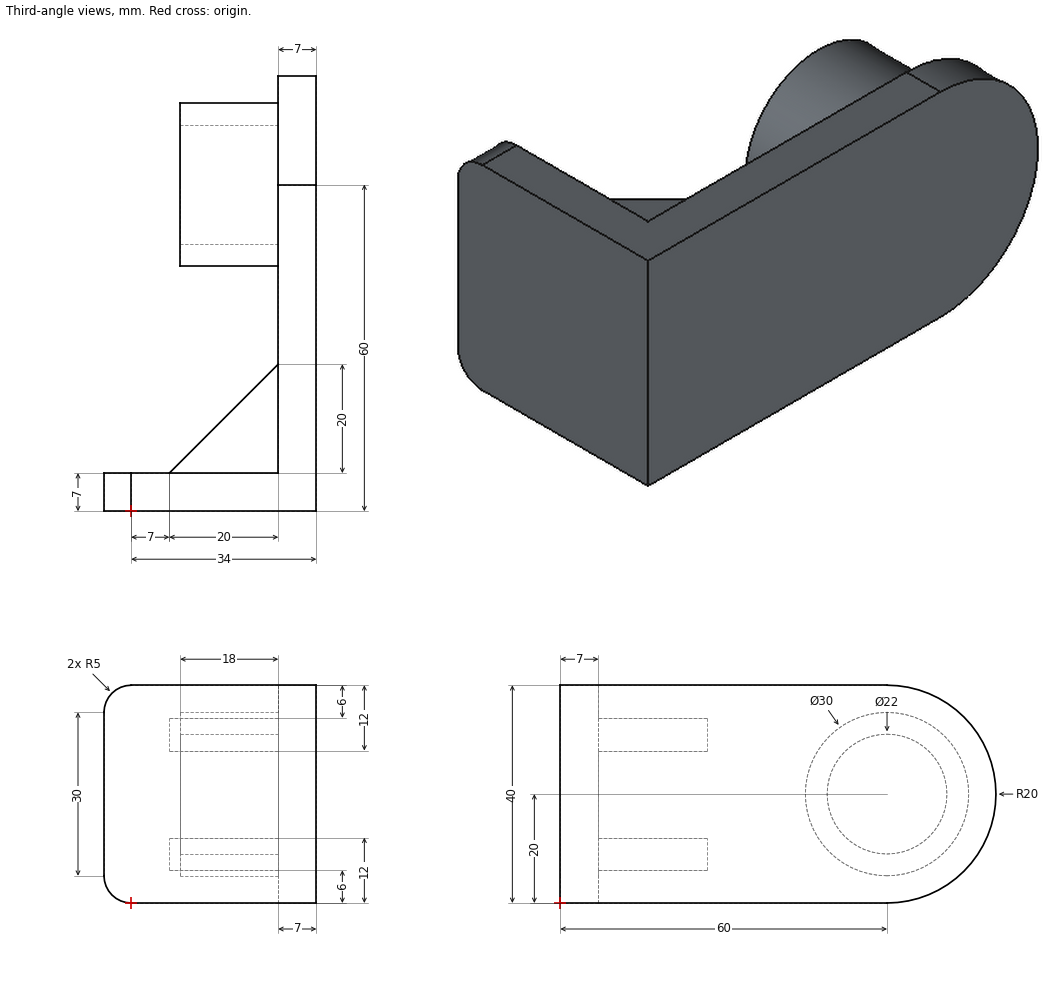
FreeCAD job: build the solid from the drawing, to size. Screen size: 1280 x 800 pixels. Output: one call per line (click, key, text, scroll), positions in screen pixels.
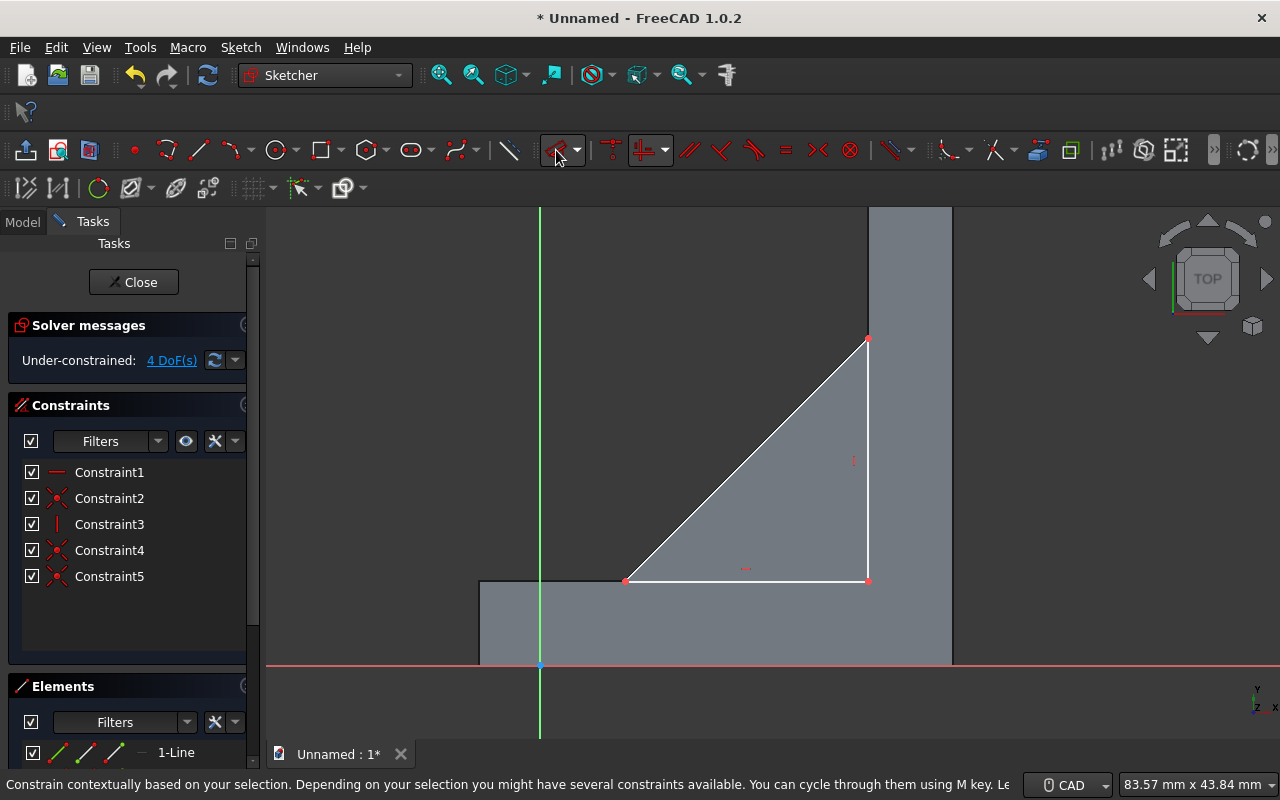
click(698, 582)
click(747, 616)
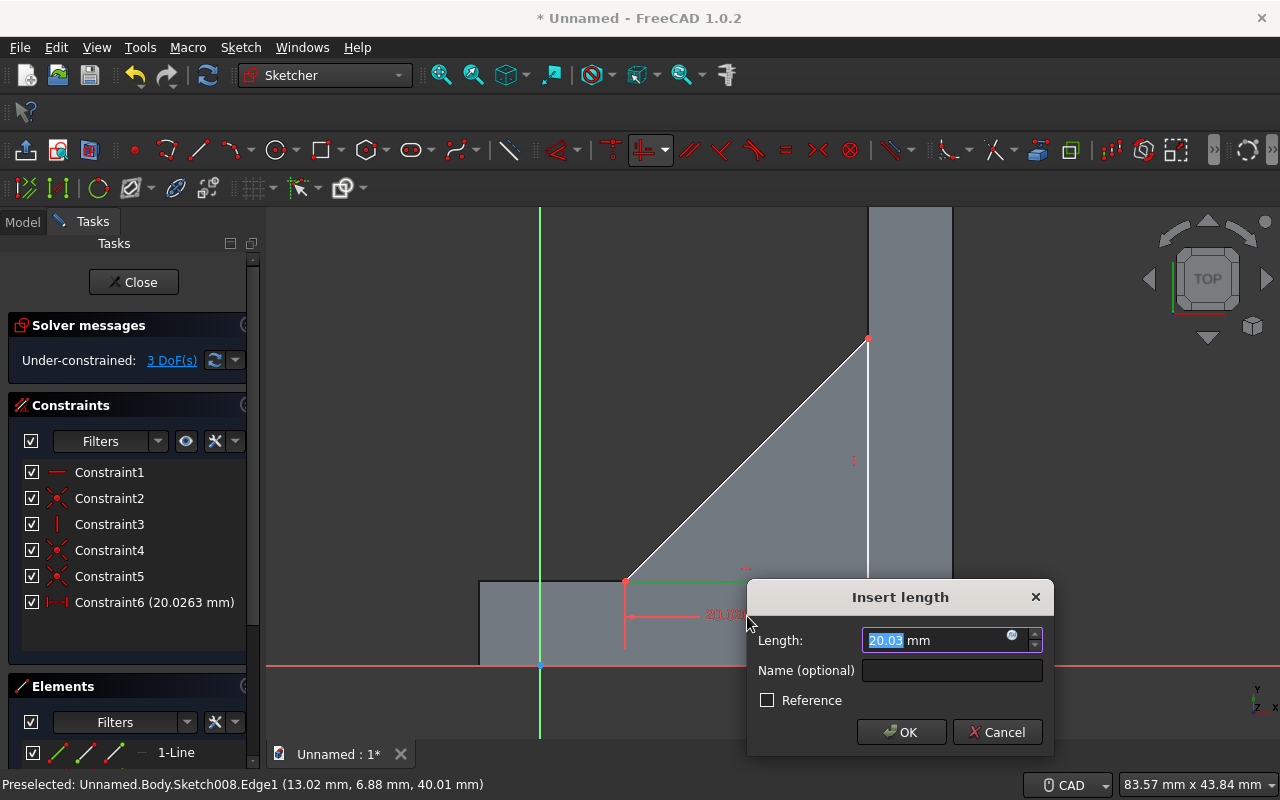
text(20)
key(Return)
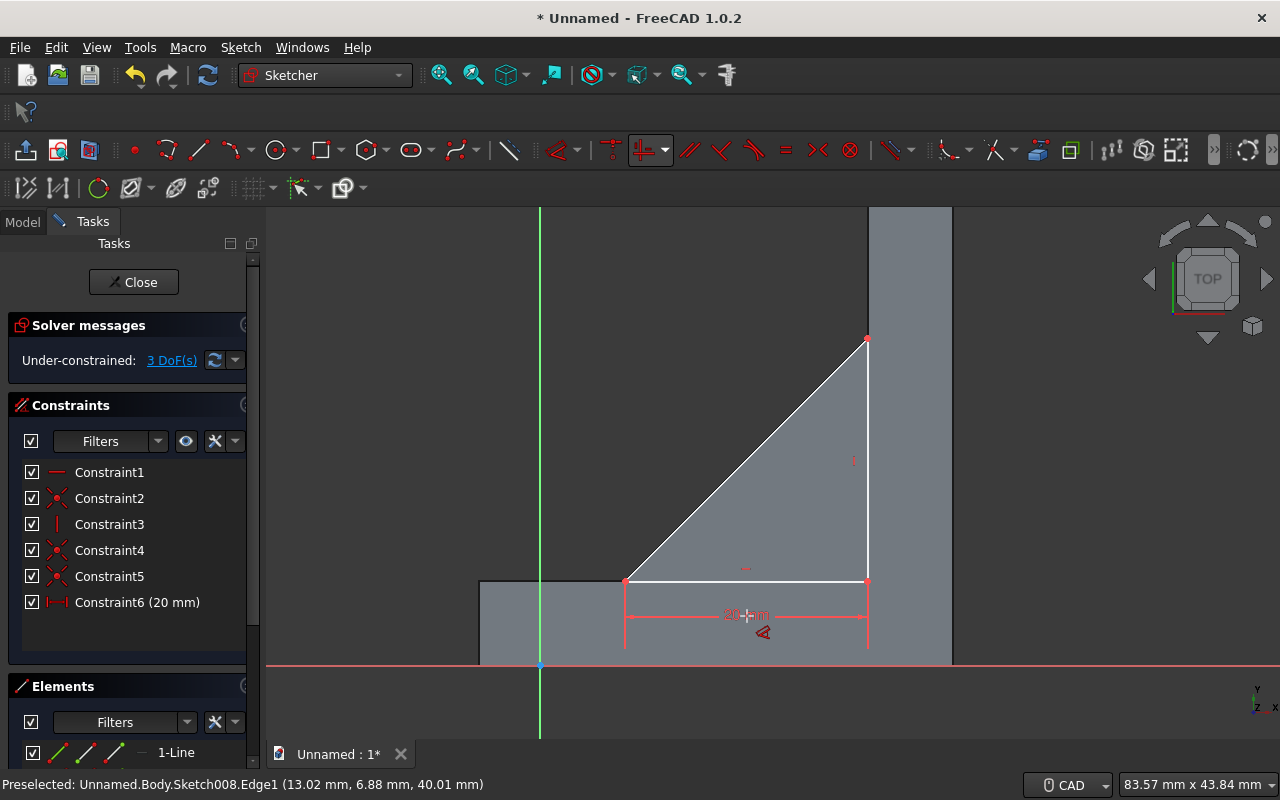
click(868, 509)
click(902, 461)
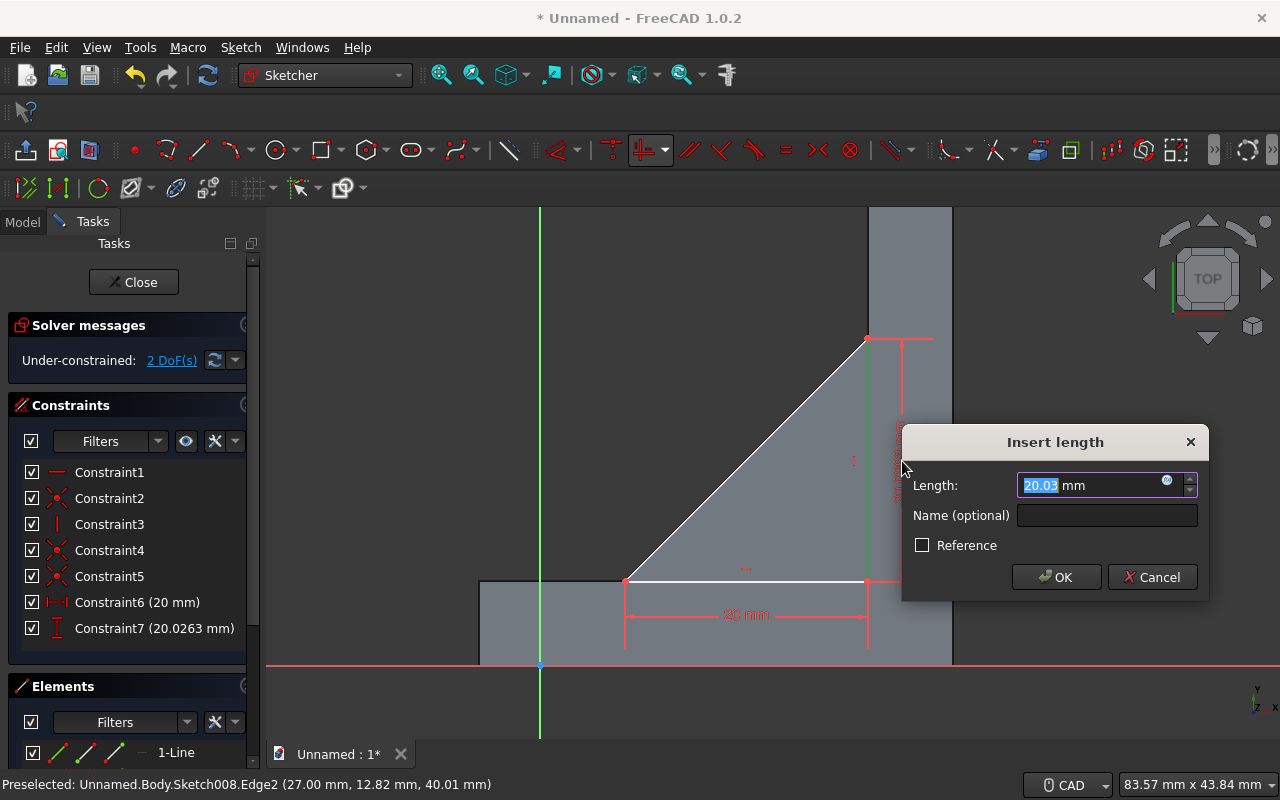
text(20)
key(Return)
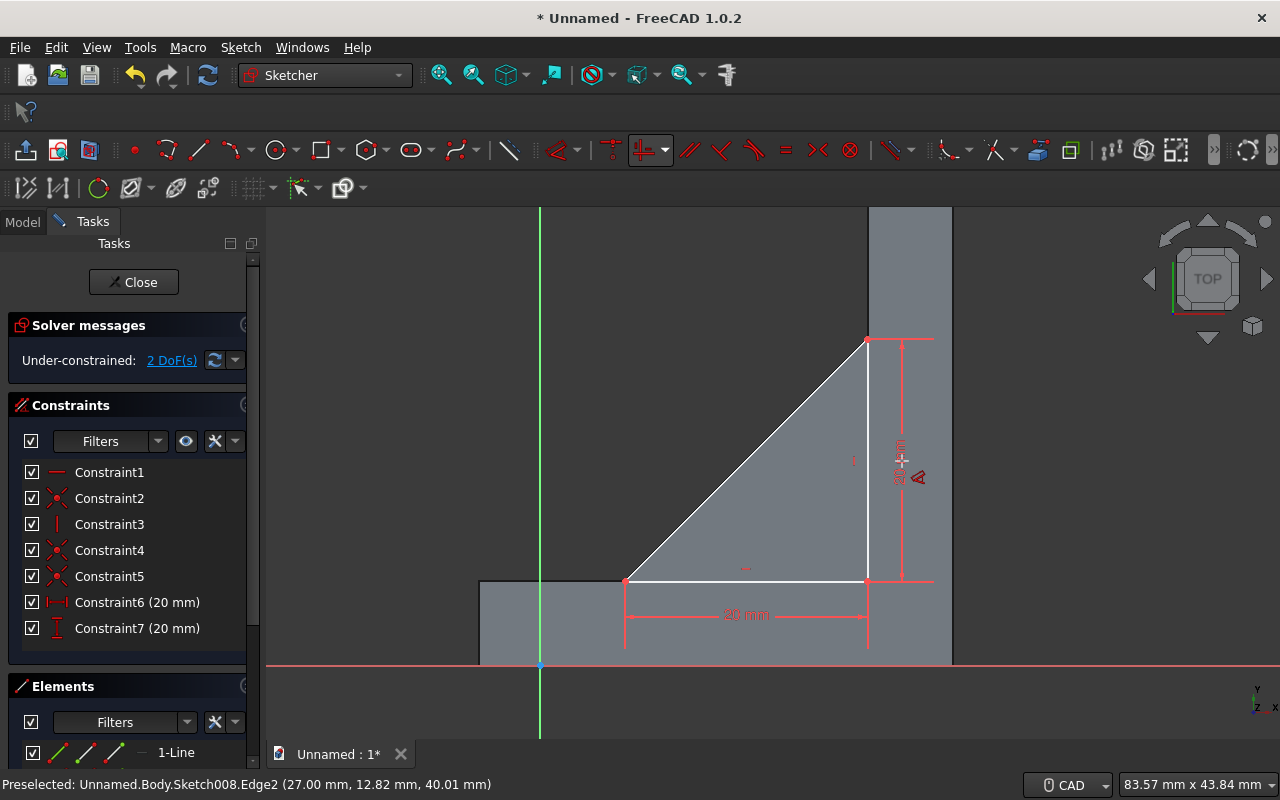
click(625, 582)
click(583, 700)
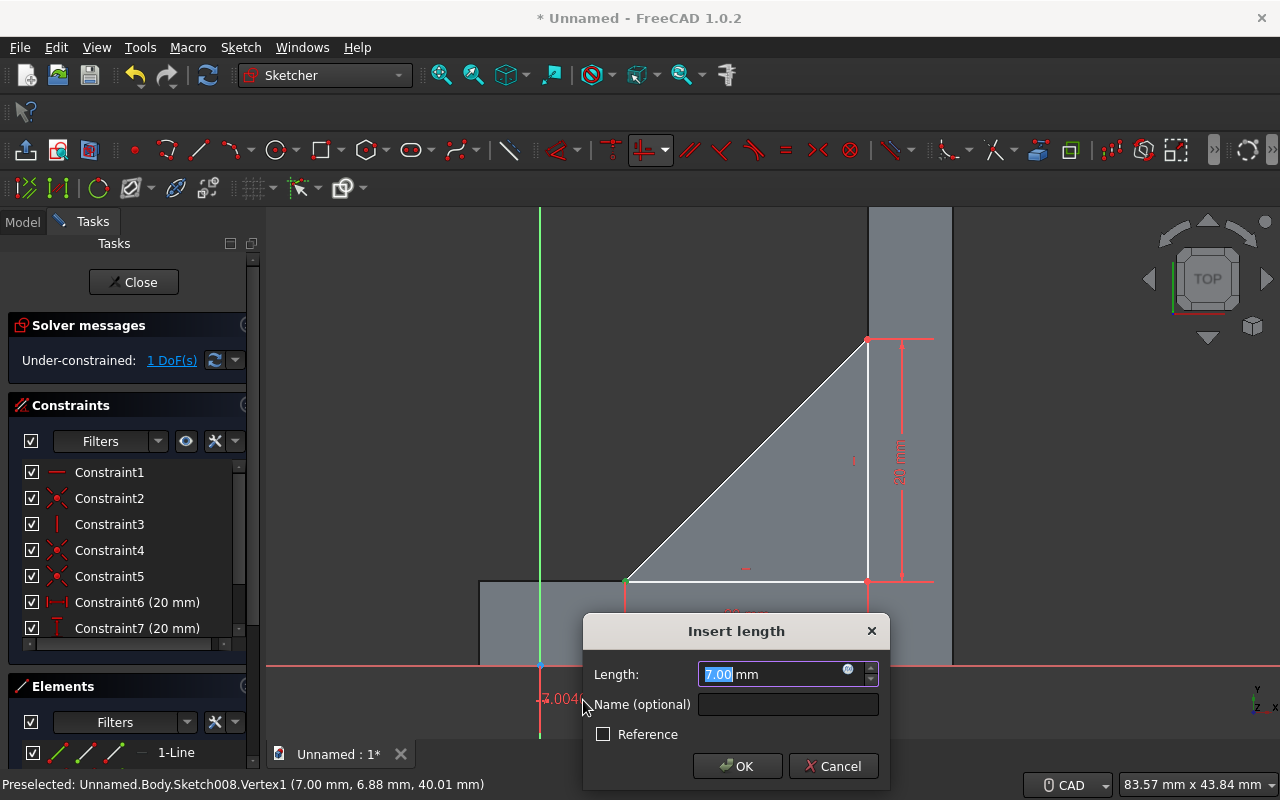
text(7)
key(Return)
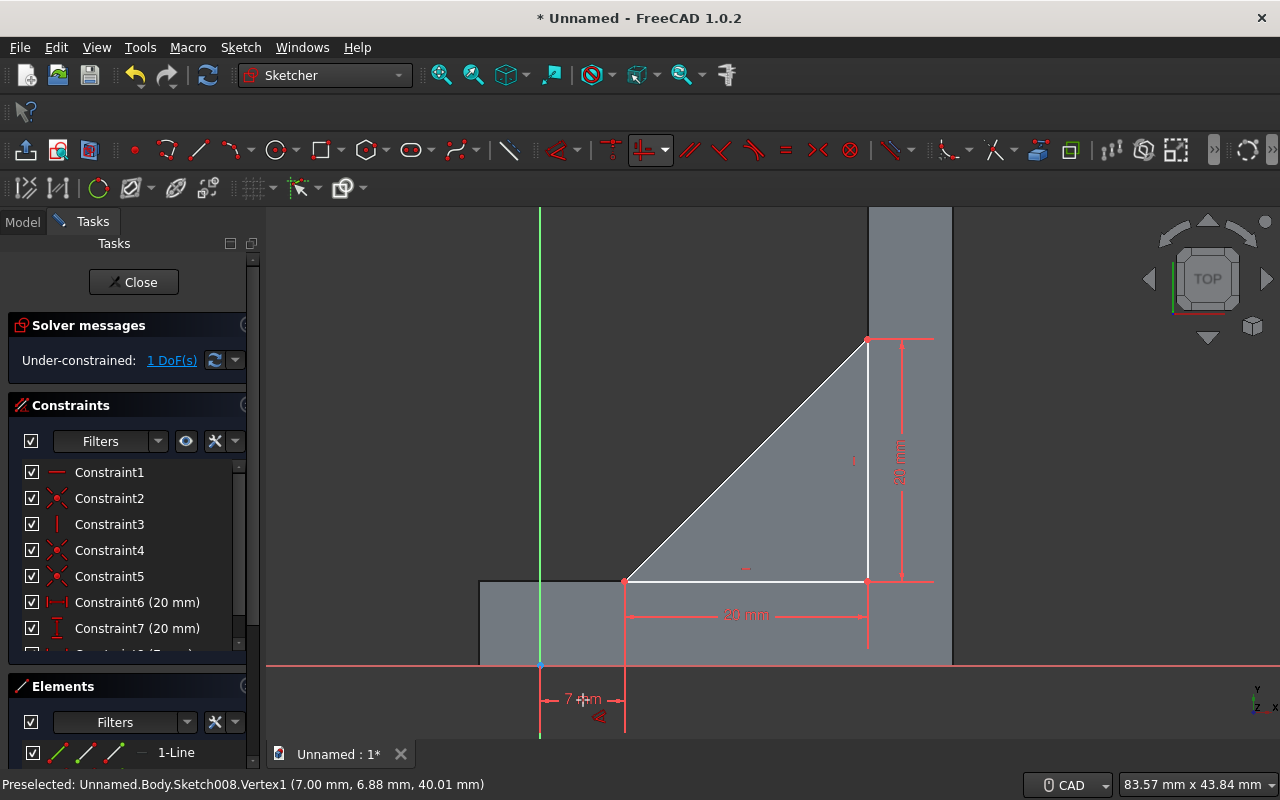
click(625, 582)
click(506, 624)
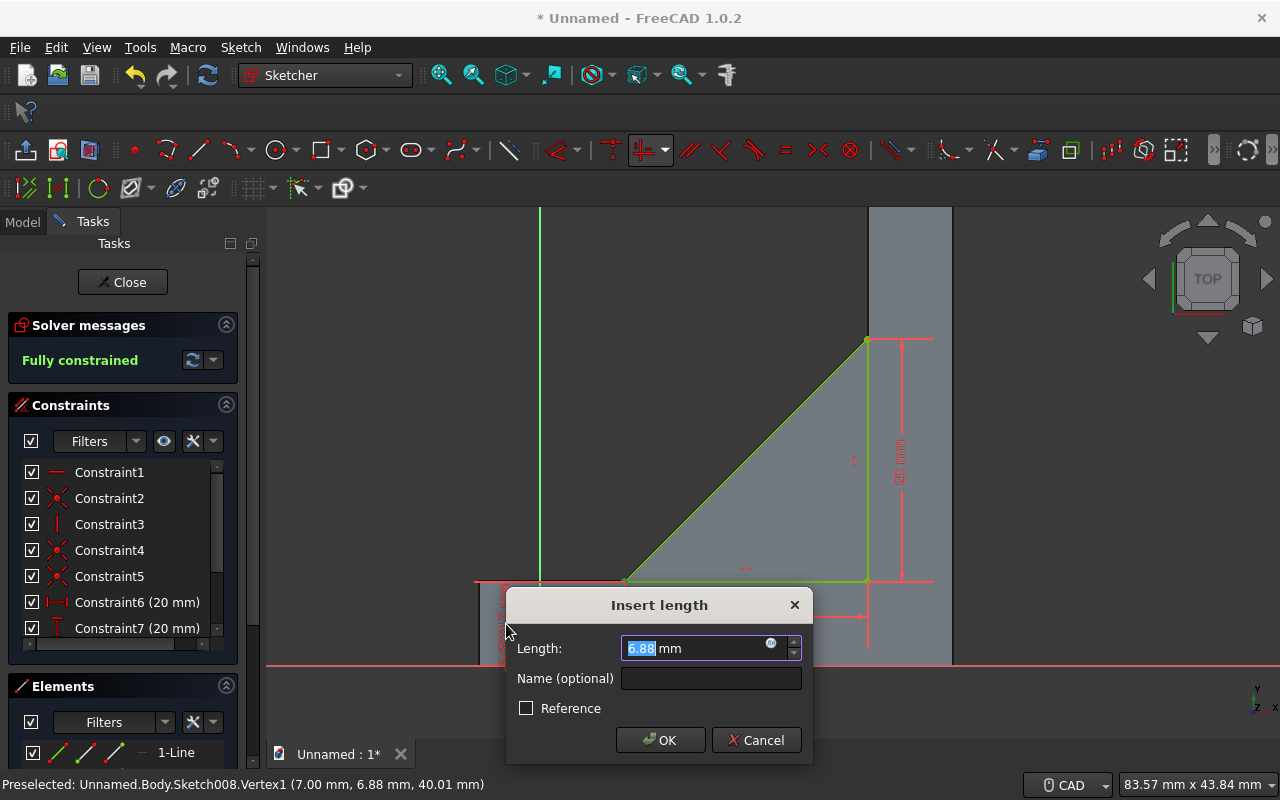
text(7)
key(Return)
key(Escape)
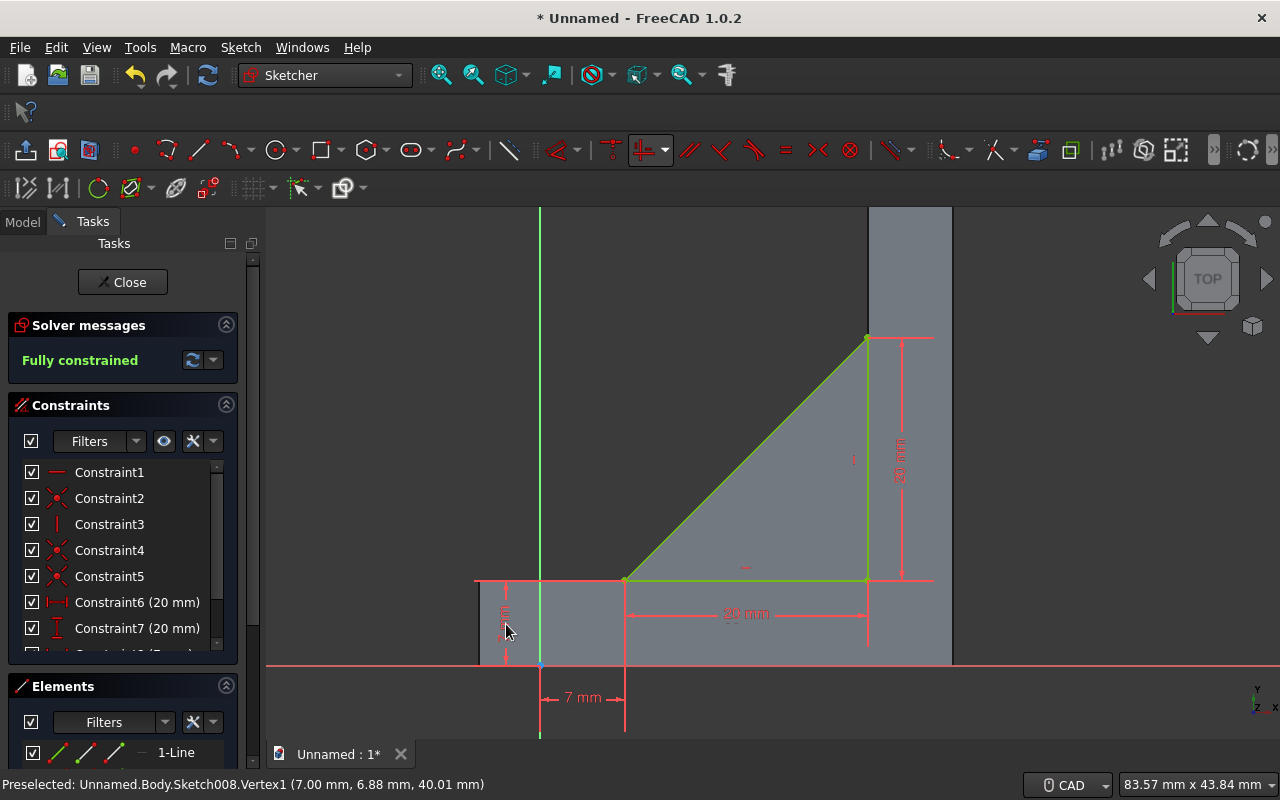
click(123, 282)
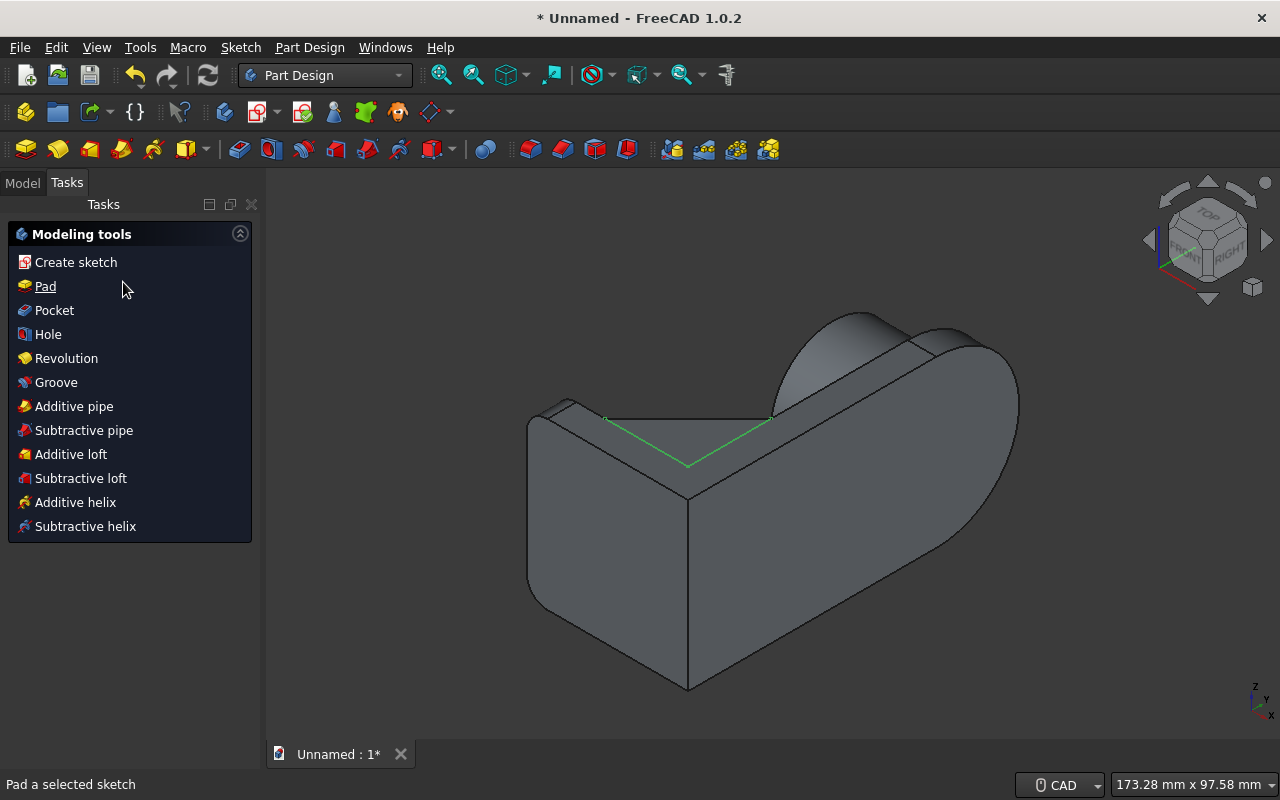
click(240, 150)